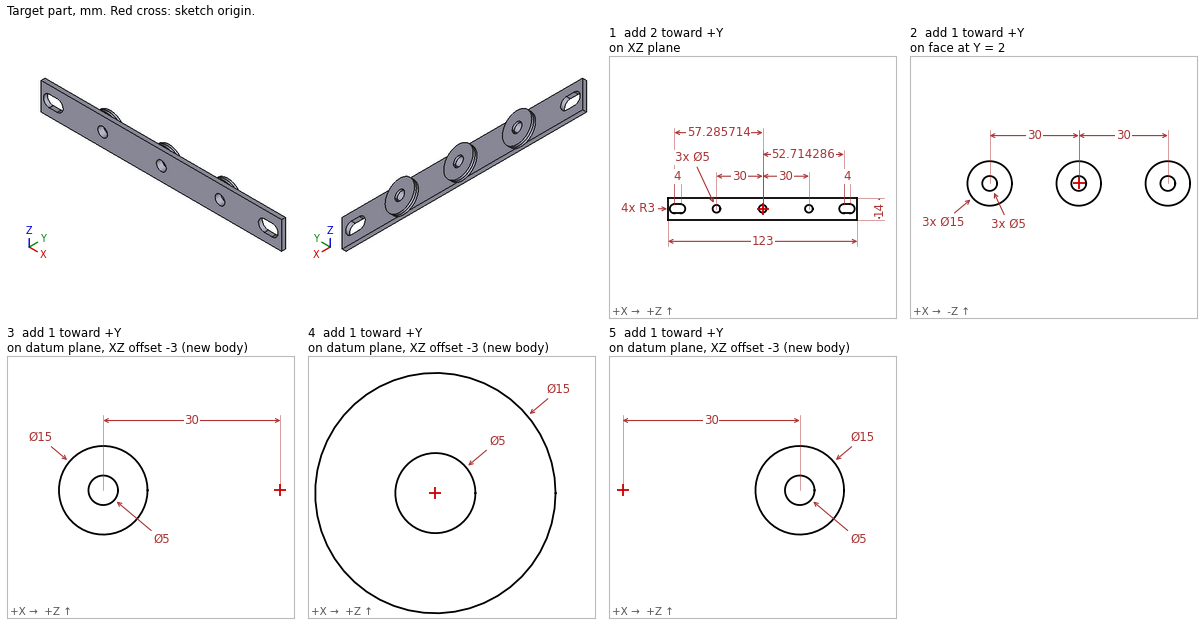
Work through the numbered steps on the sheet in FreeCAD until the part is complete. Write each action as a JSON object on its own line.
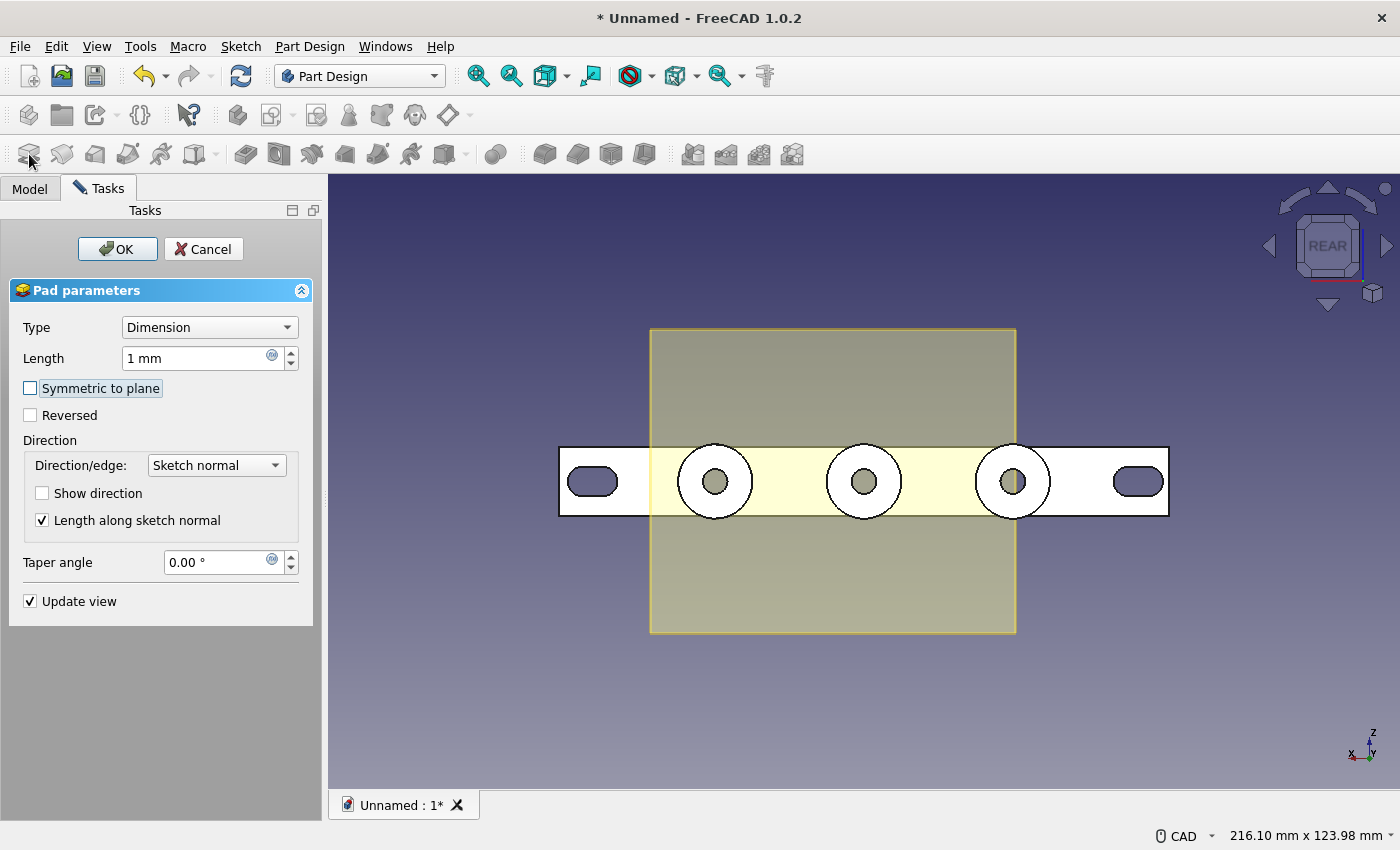
{"action": "left_click", "coordinate": [31, 415]}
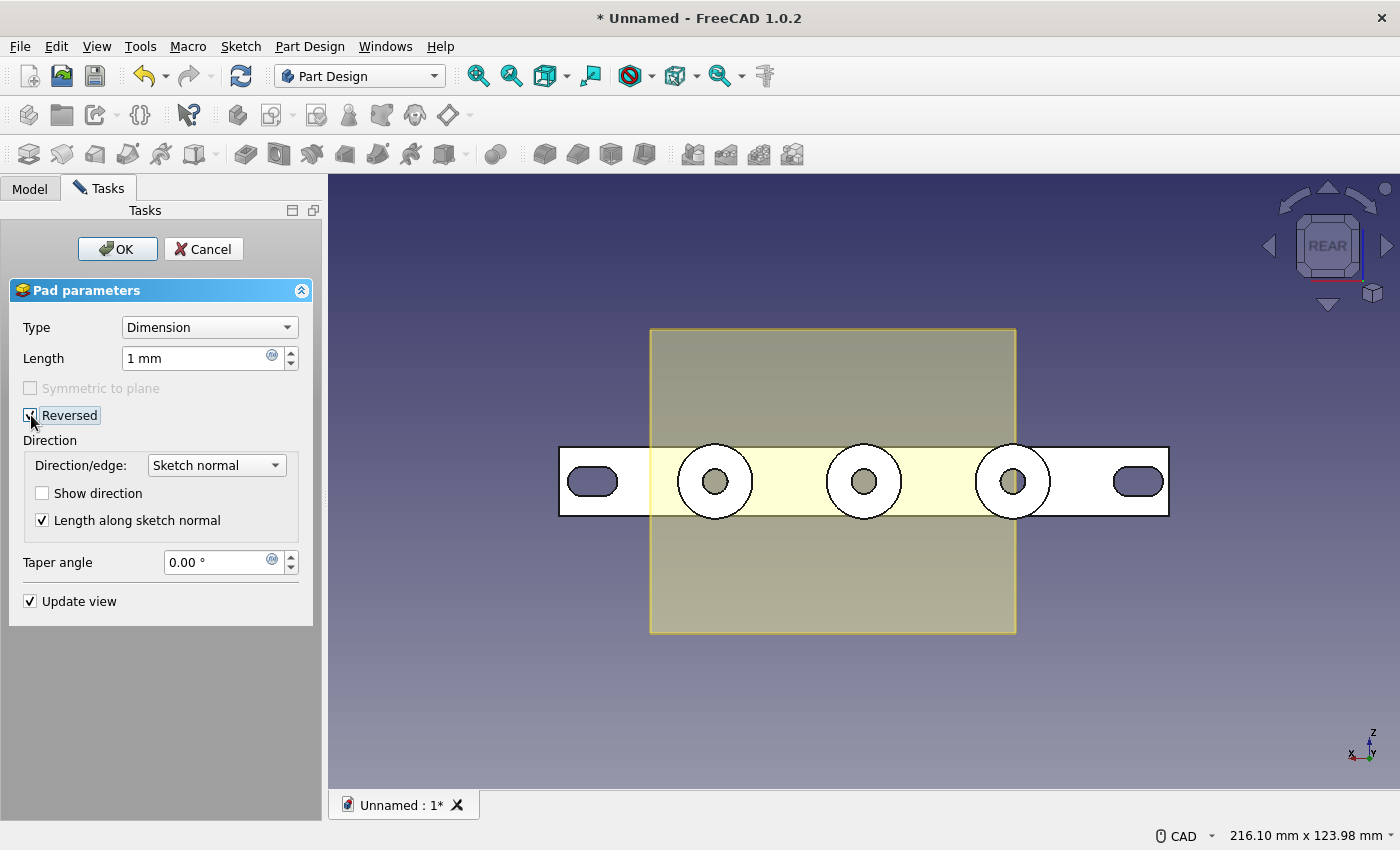
{"action": "left_click", "coordinate": [118, 249]}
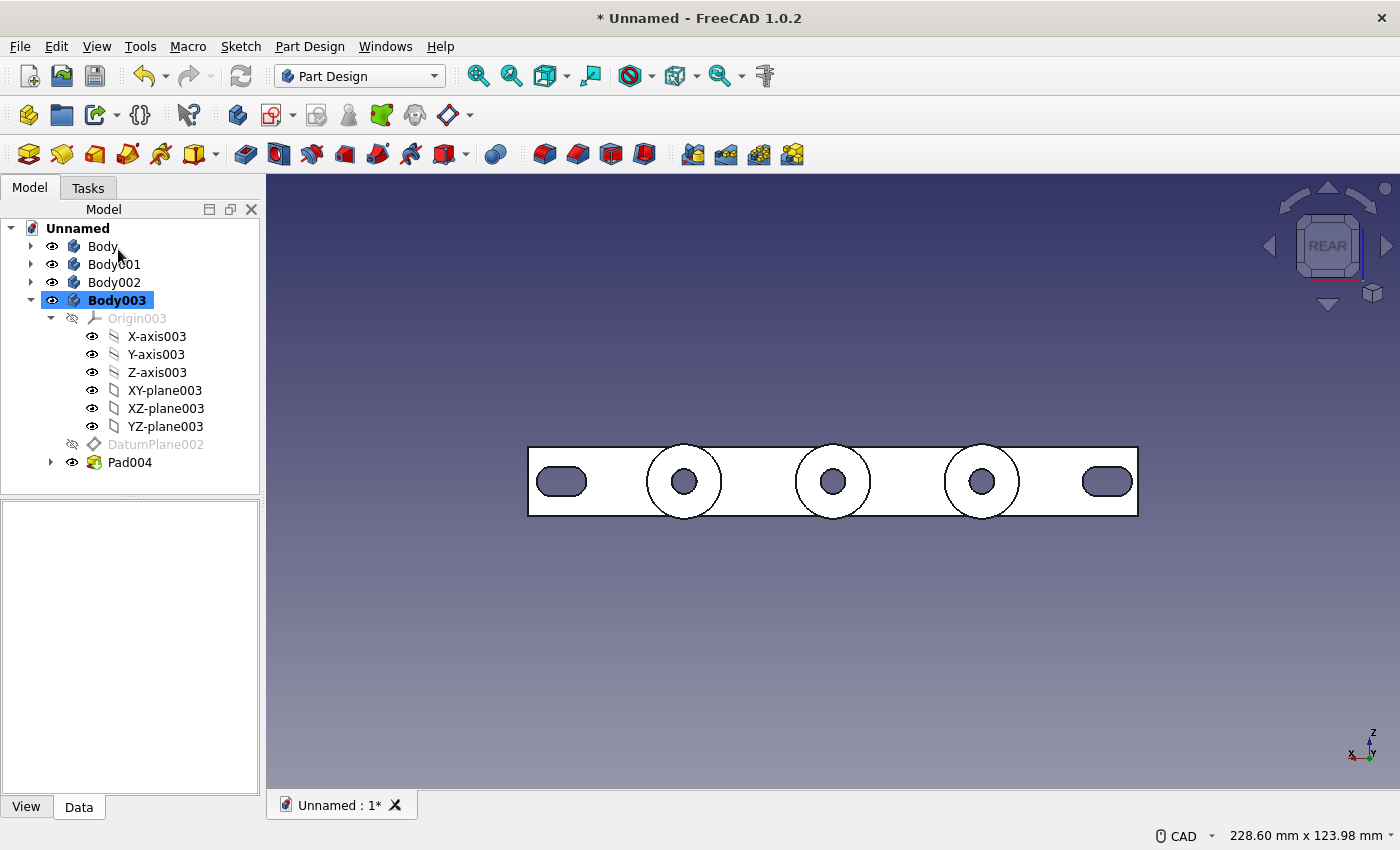
{"action": "key", "text": "0"}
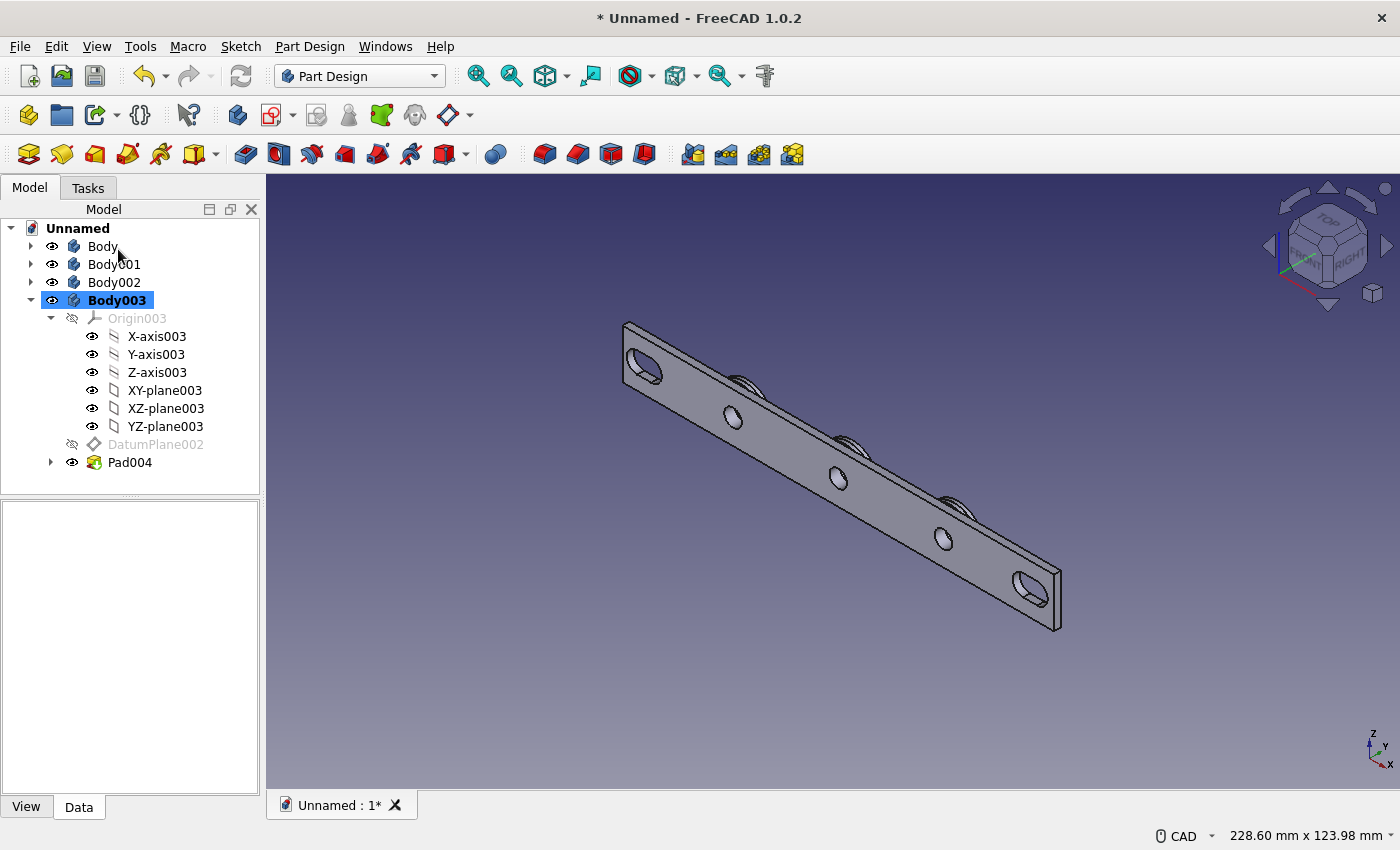
{"action": "left_click", "coordinate": [479, 76]}